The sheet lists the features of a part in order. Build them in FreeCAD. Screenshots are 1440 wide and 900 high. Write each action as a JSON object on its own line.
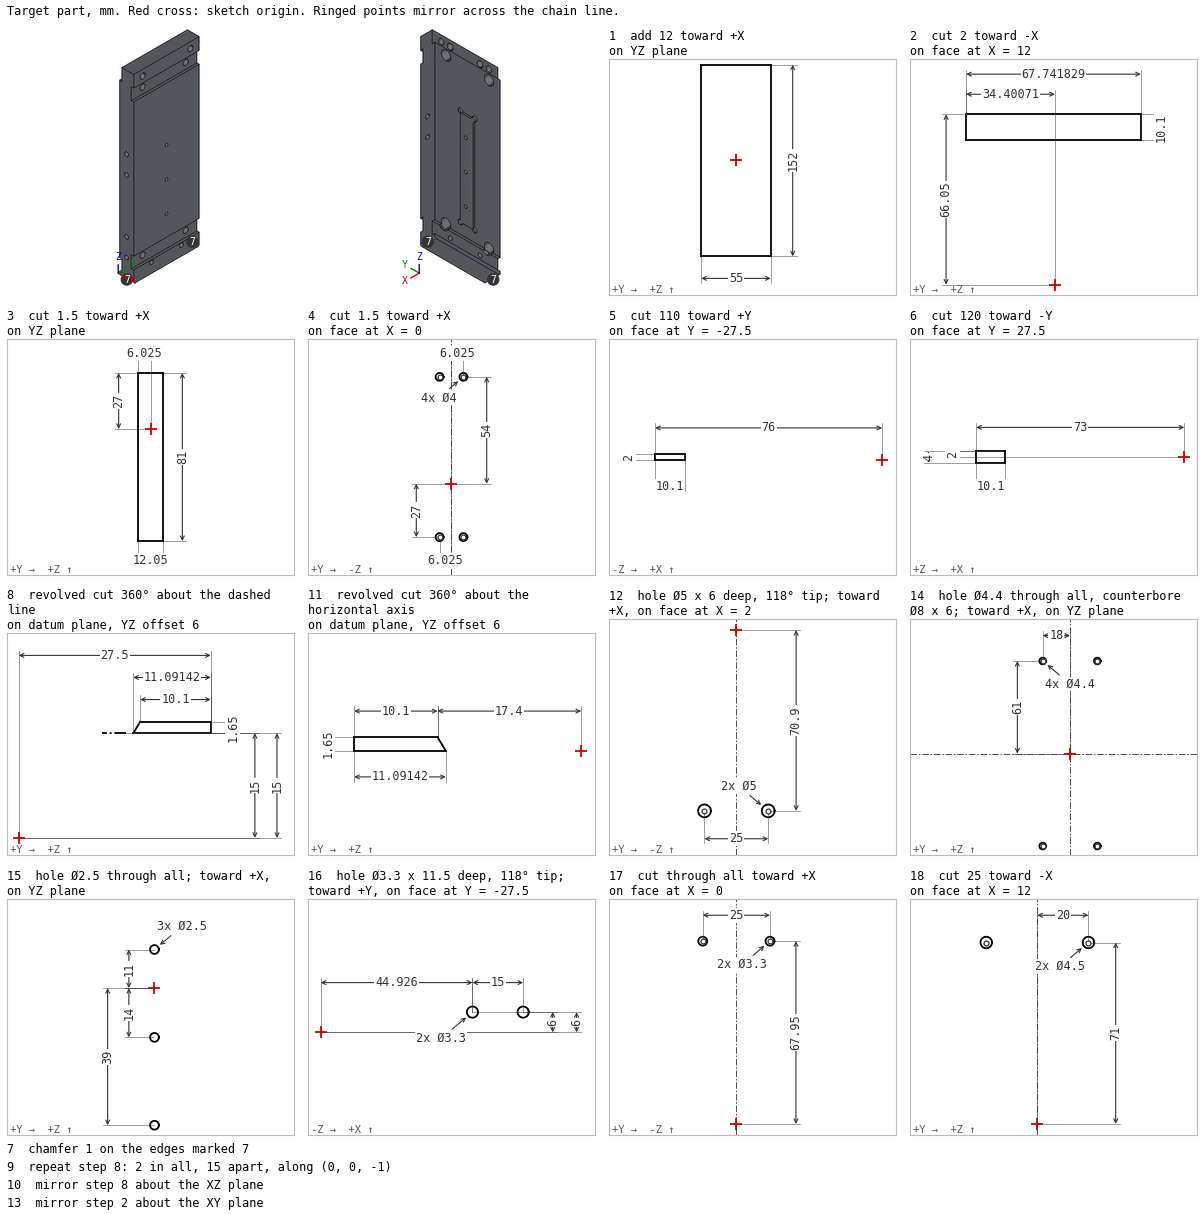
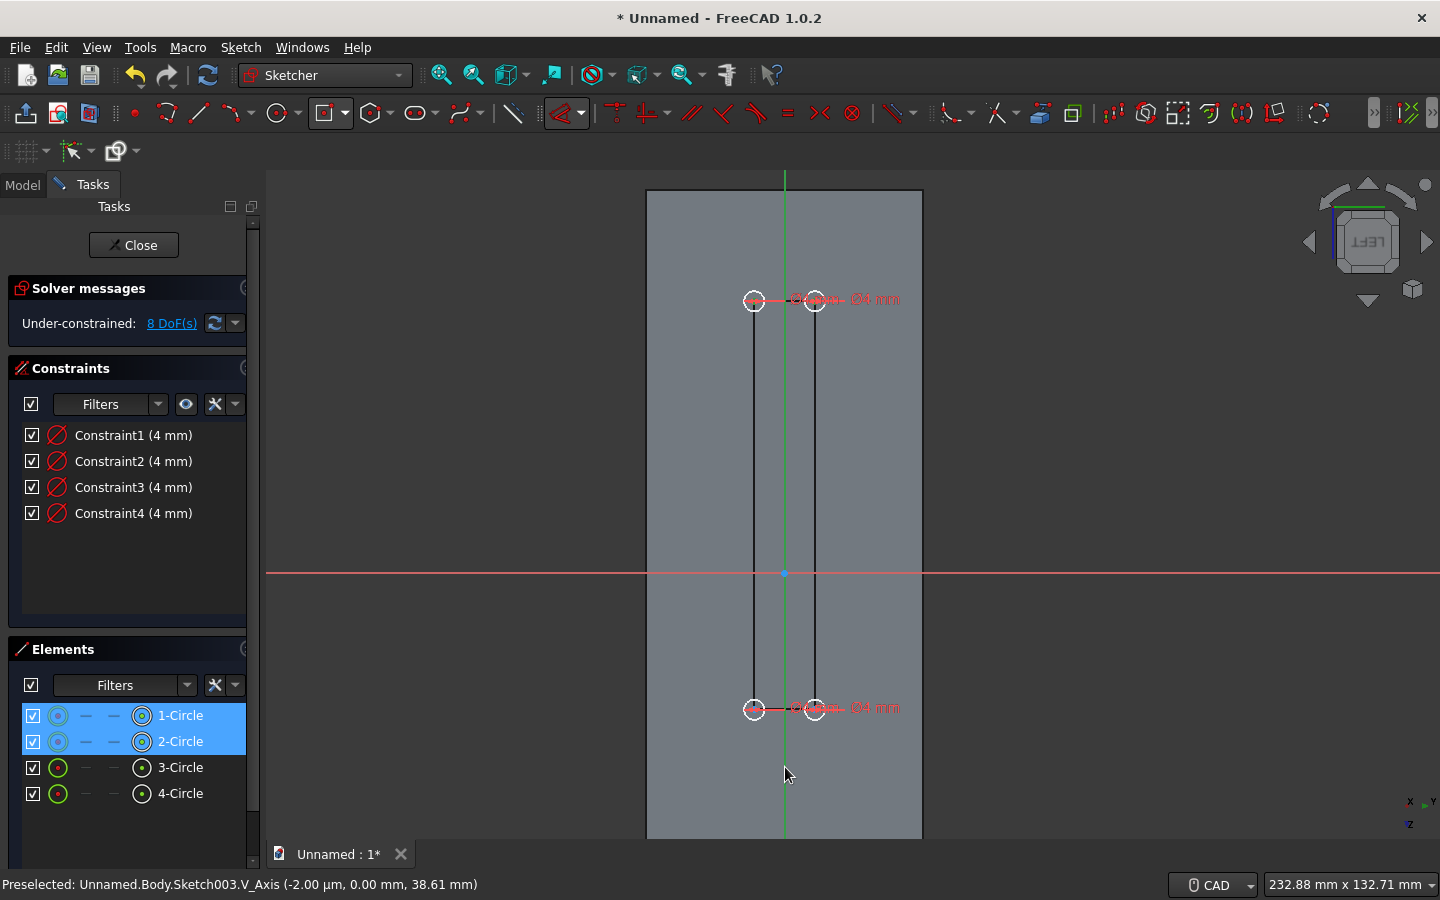
{"action": "left_click", "coordinate": [820, 114]}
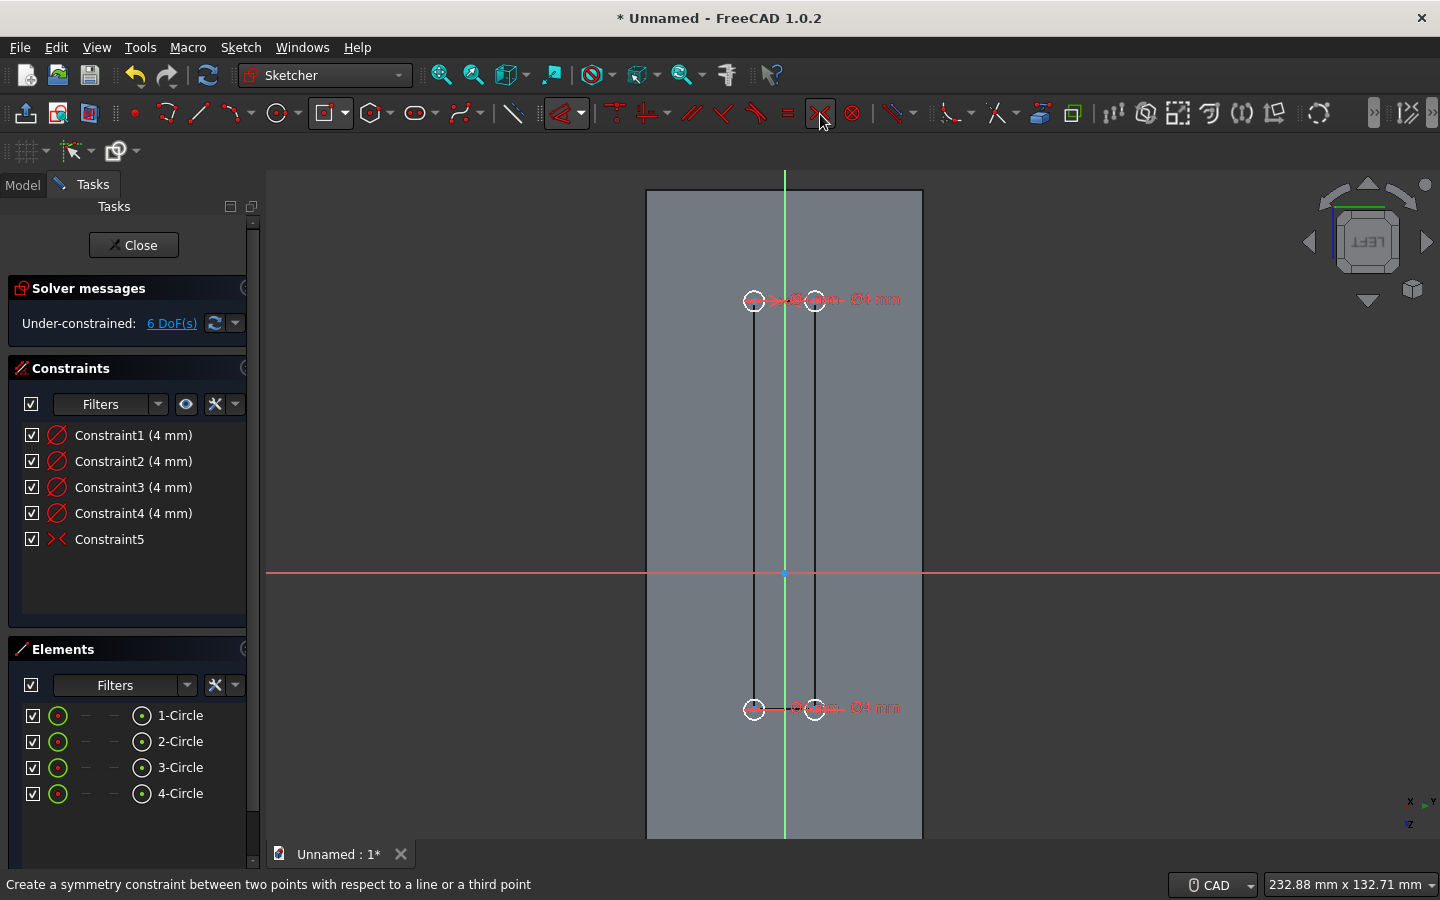
{"action": "left_click", "coordinate": [754, 710]}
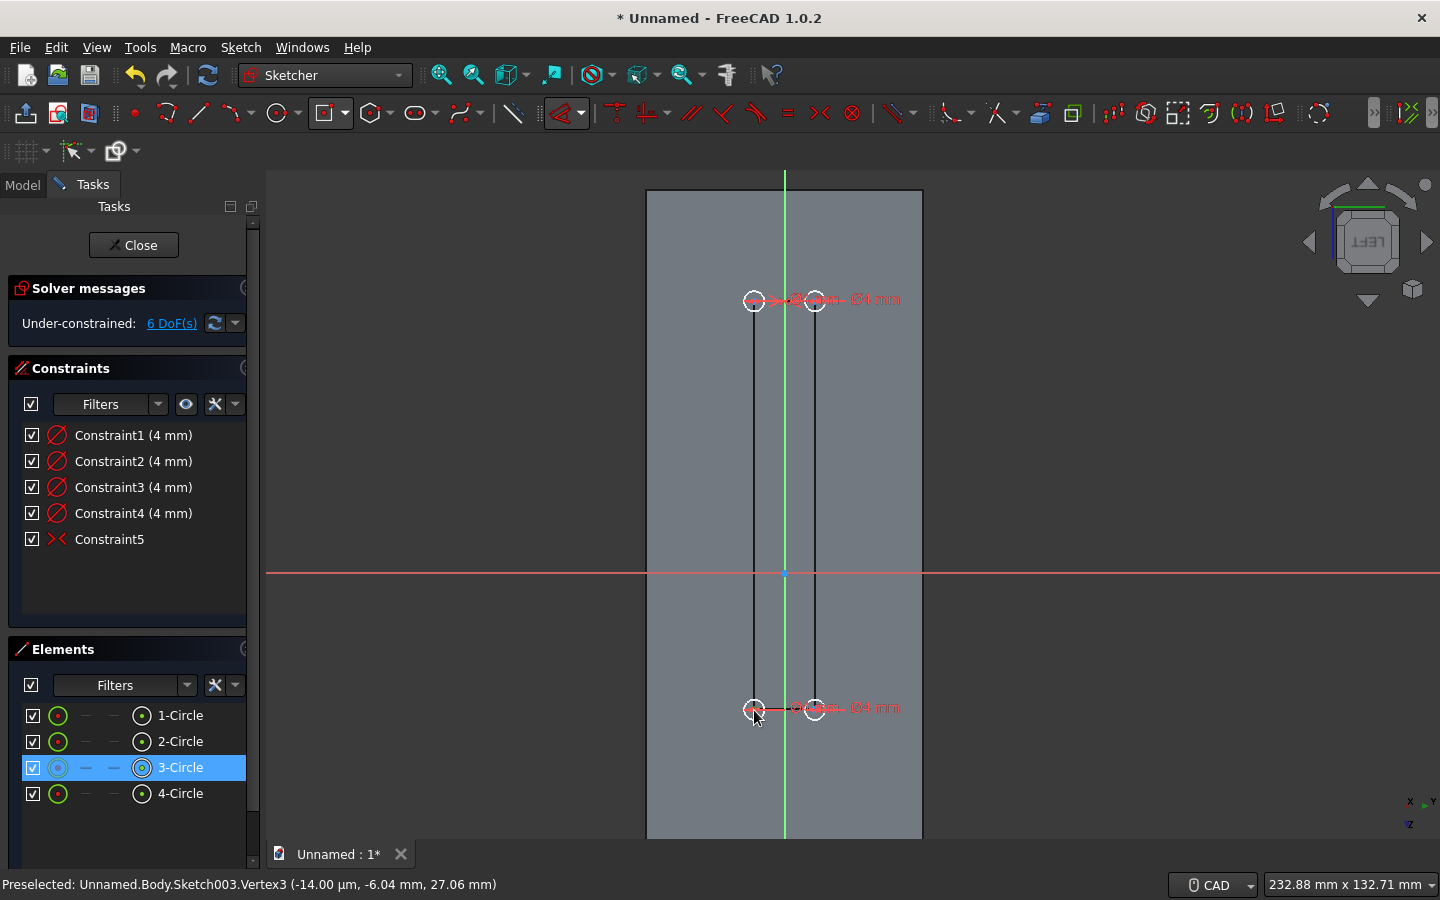
{"action": "left_click", "coordinate": [815, 710]}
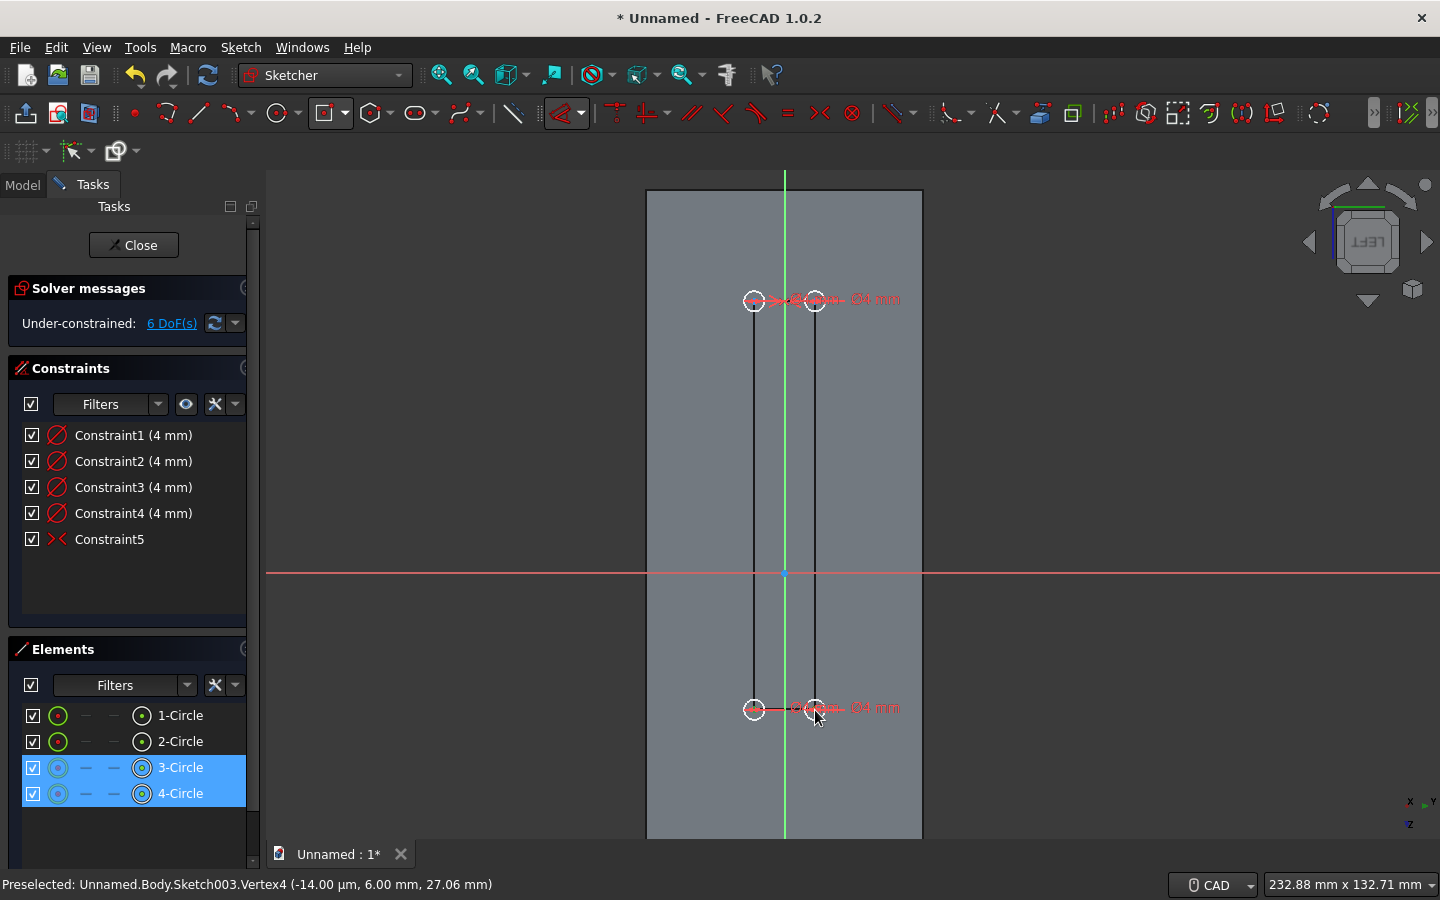
{"action": "left_click", "coordinate": [785, 767]}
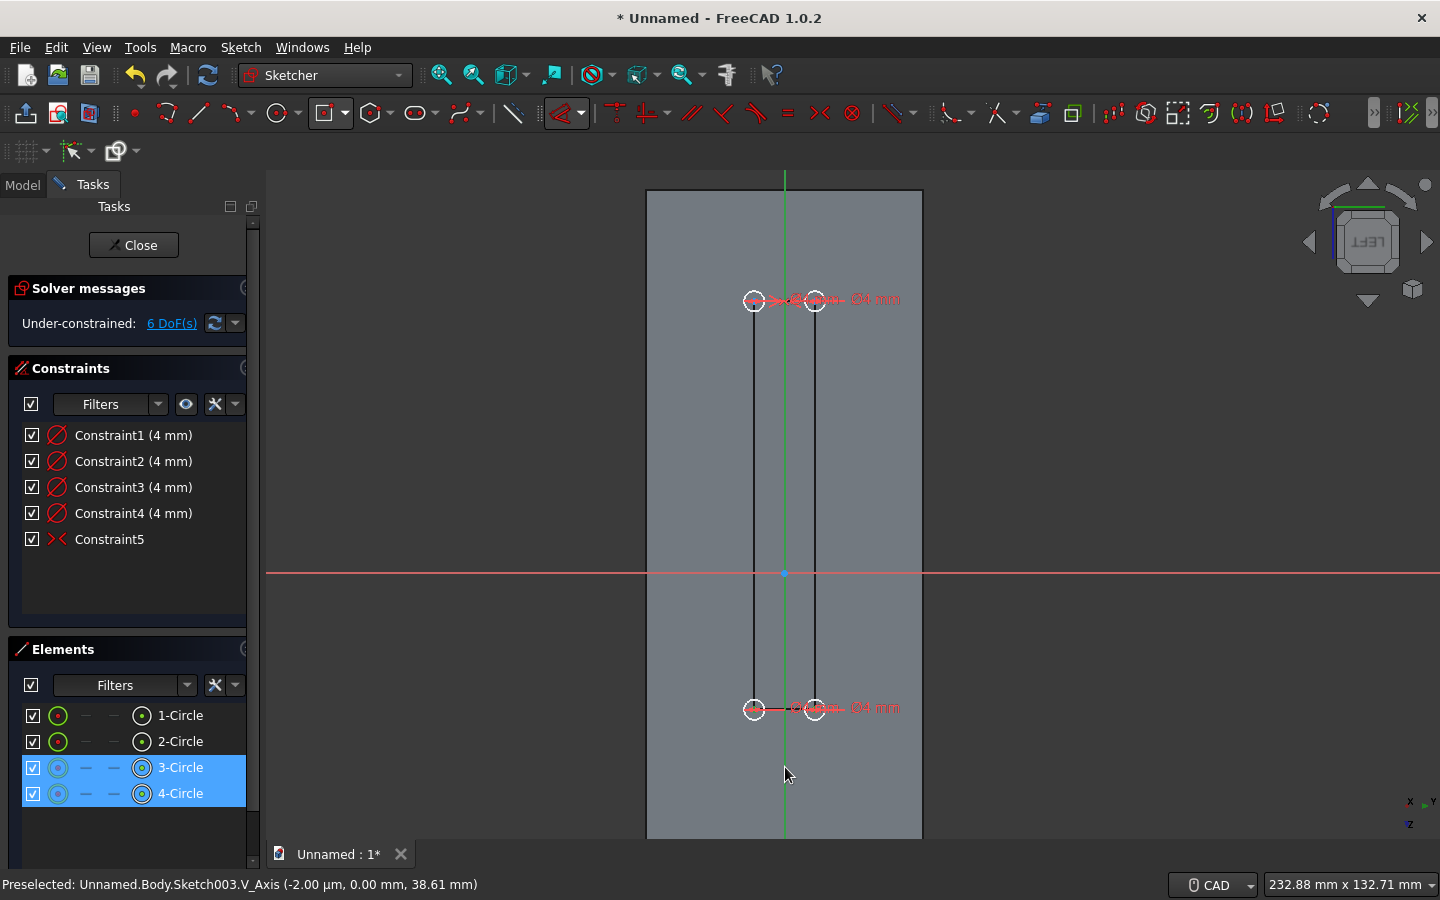
{"action": "key", "text": "s"}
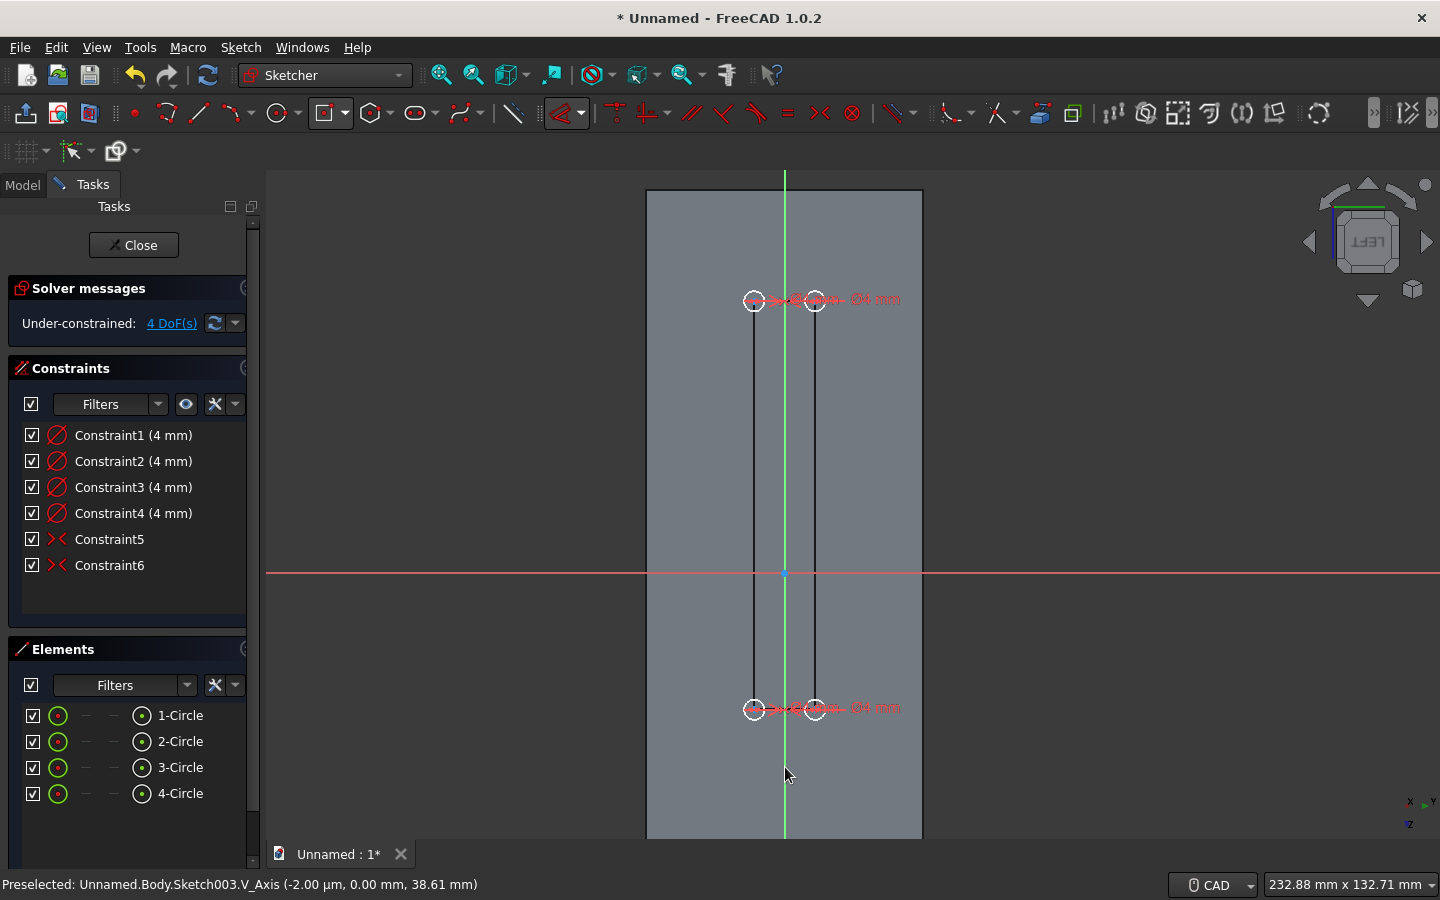
{"action": "left_click", "coordinate": [815, 301]}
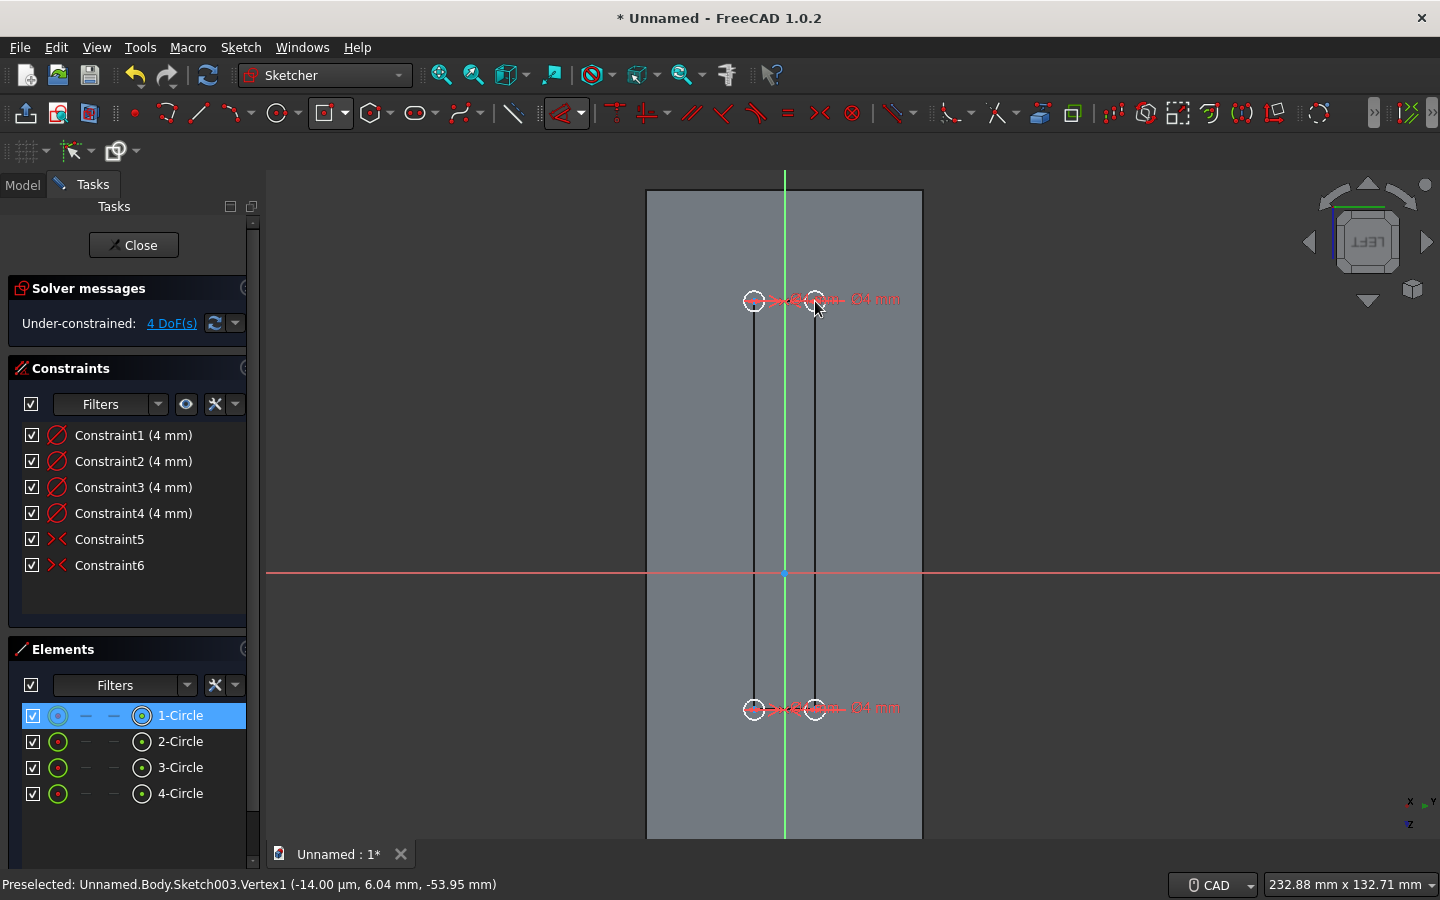
{"action": "key", "text": "i"}